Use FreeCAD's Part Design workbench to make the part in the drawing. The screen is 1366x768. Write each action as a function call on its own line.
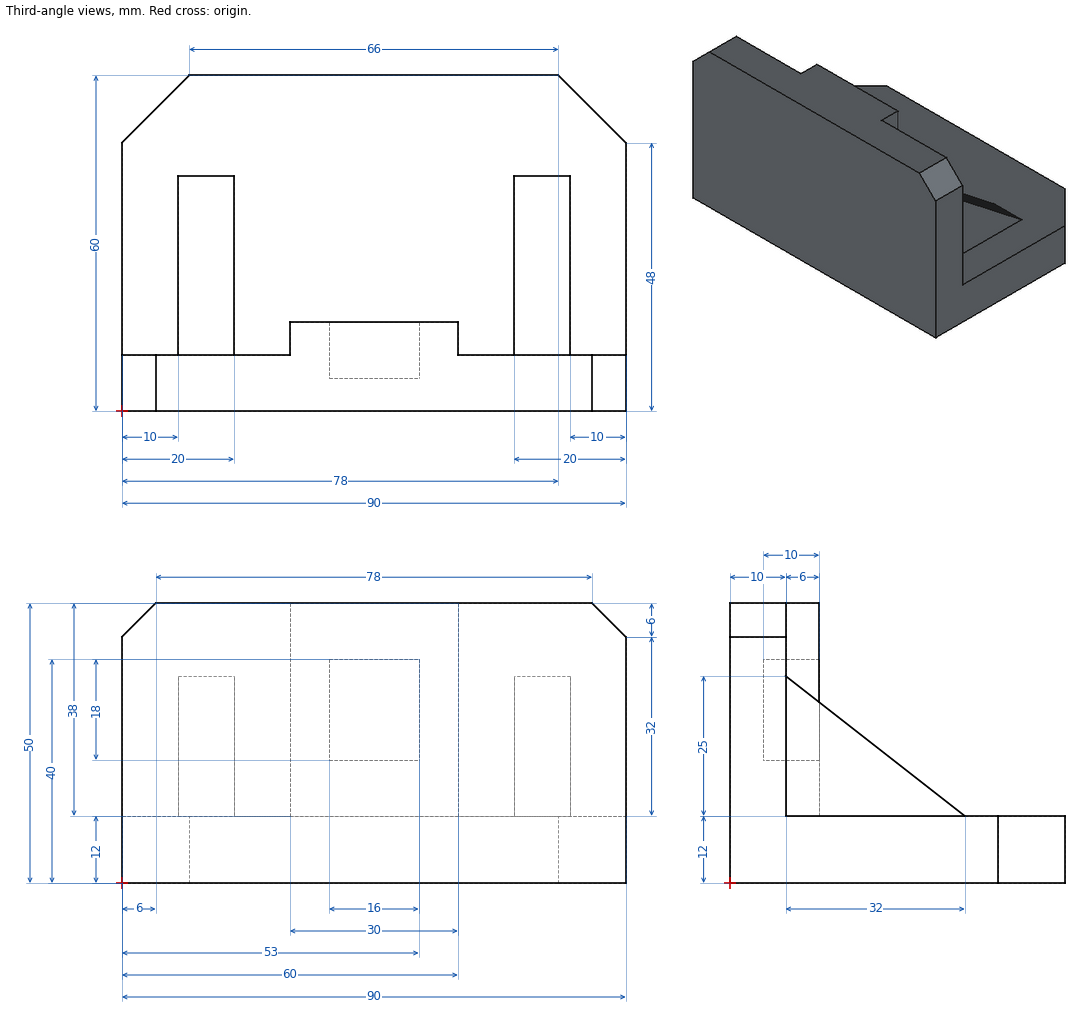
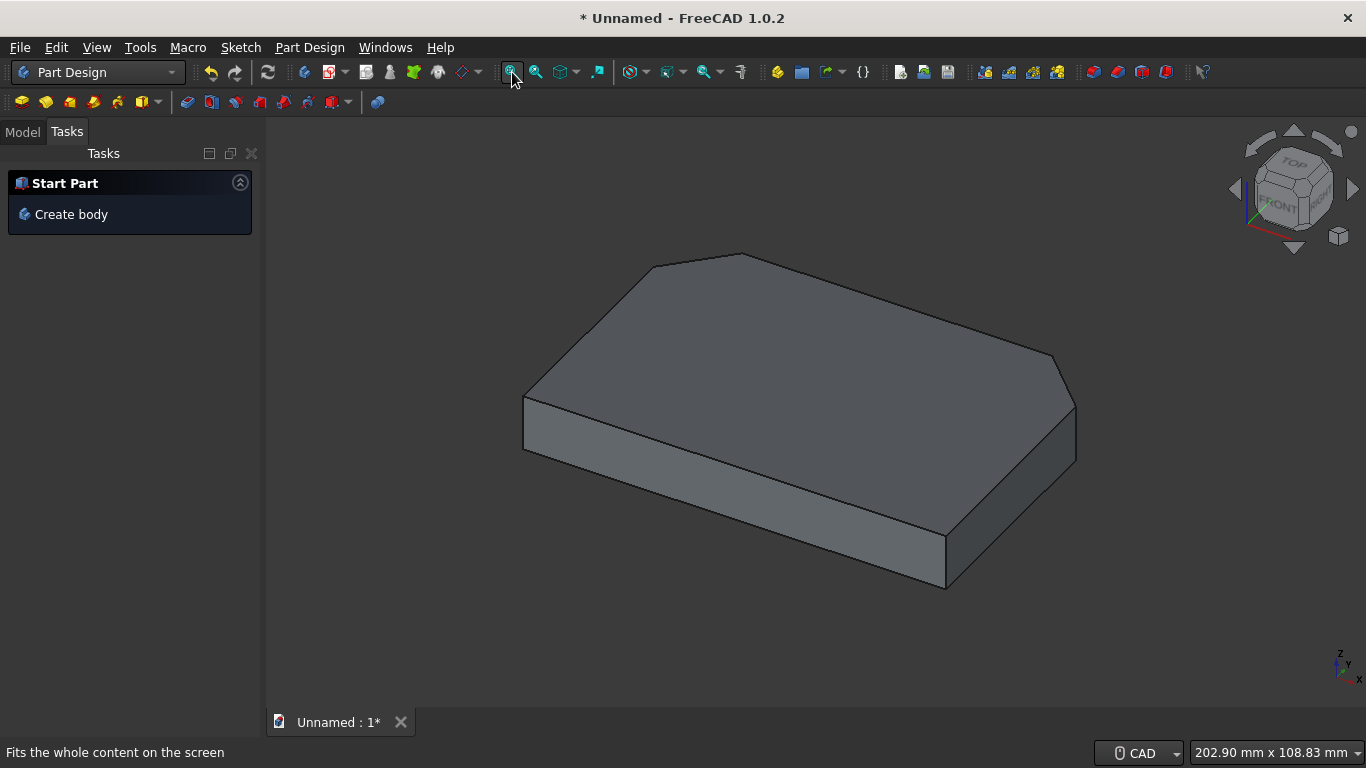
click(330, 72)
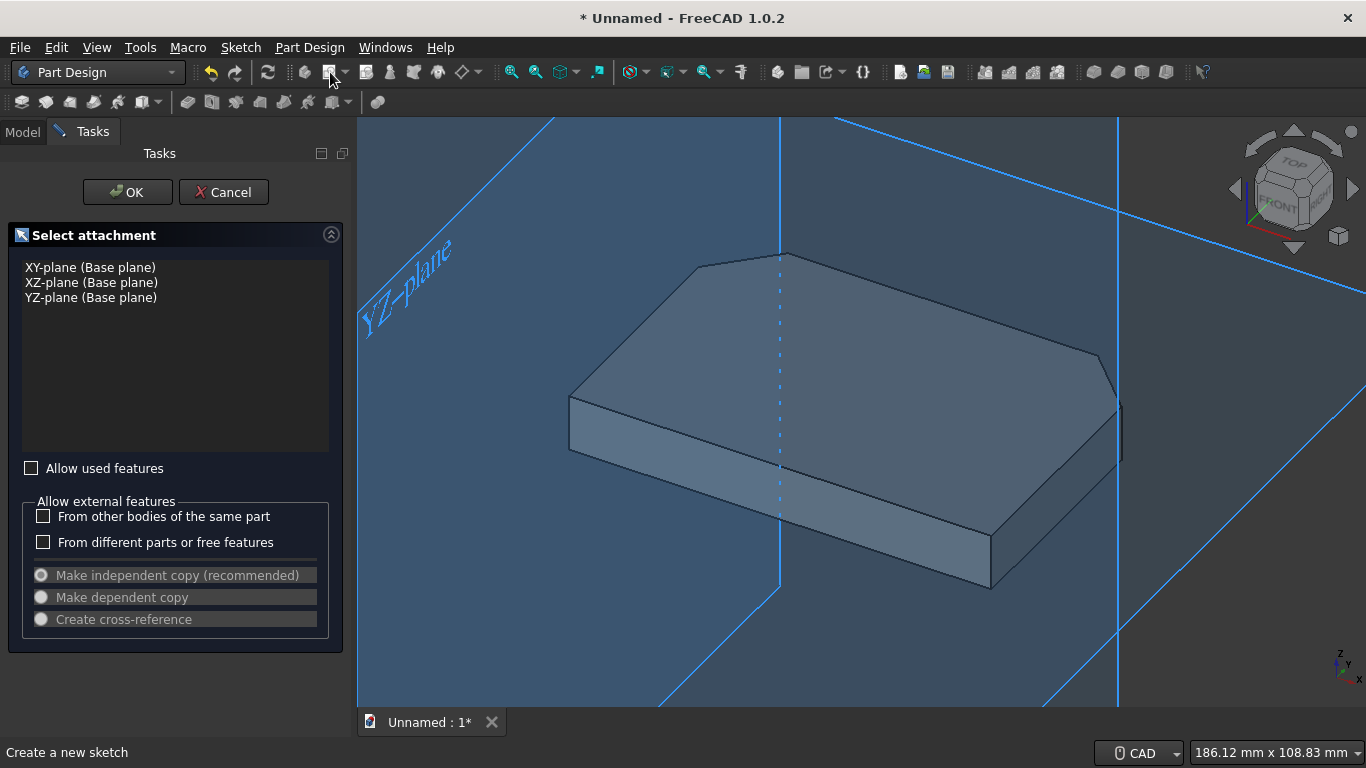
click(82, 282)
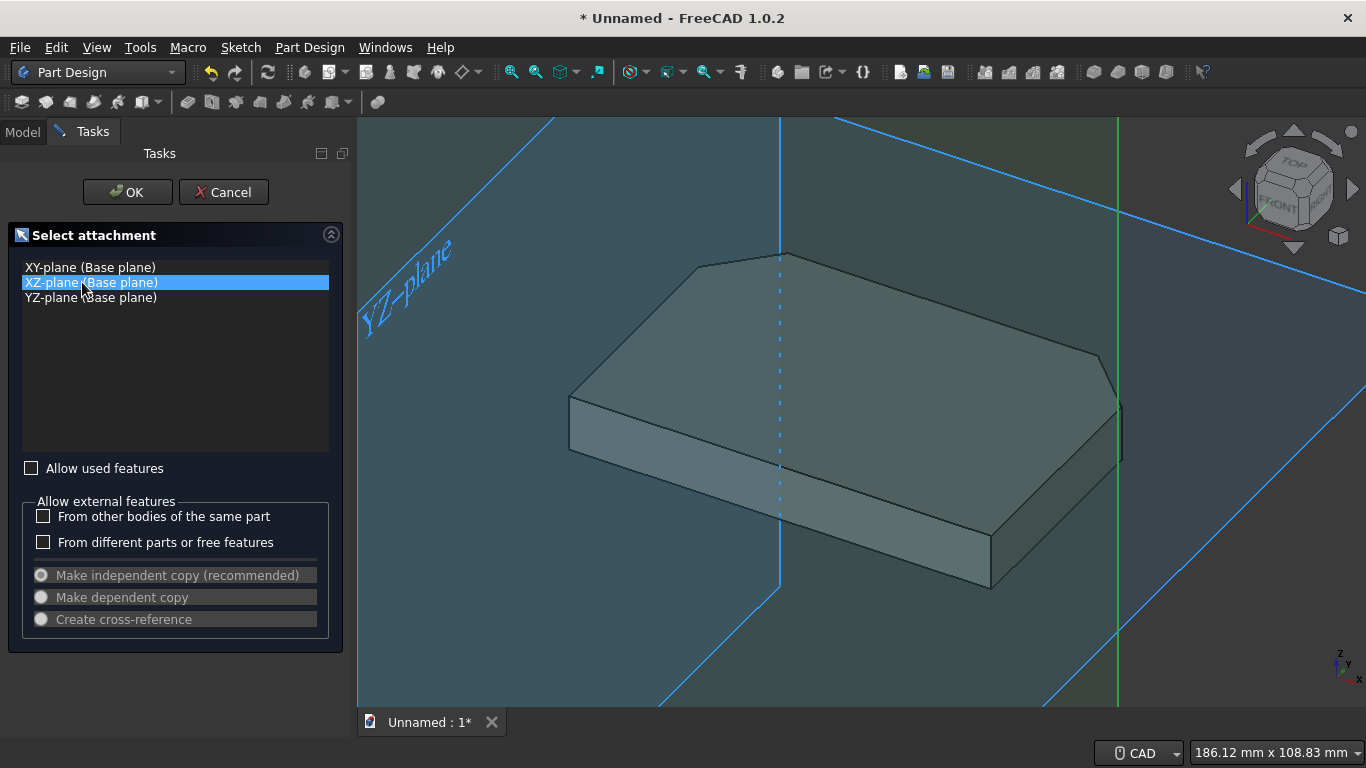
click(128, 192)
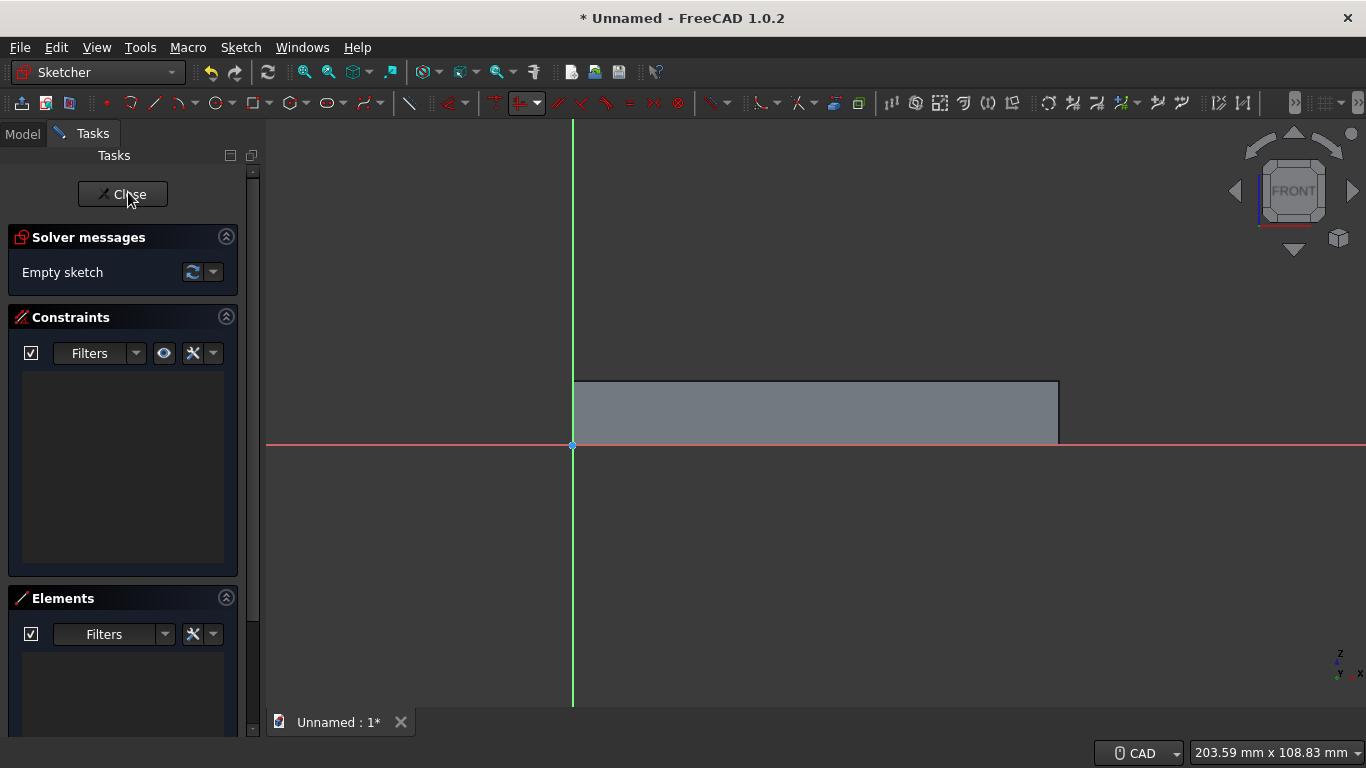
click(132, 104)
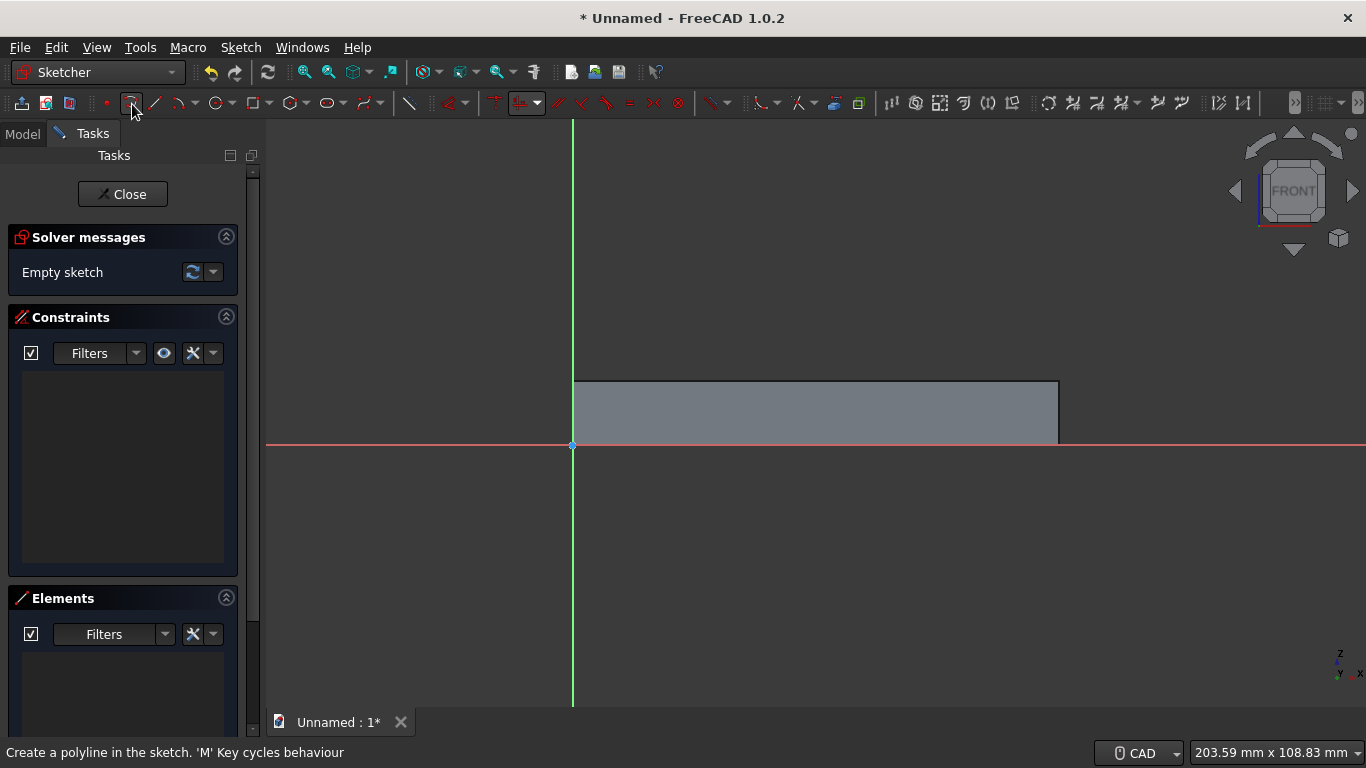
click(573, 381)
click(1059, 381)
click(1059, 208)
click(1027, 175)
click(605, 175)
click(582, 208)
click(573, 382)
key(Escape)
key(Escape)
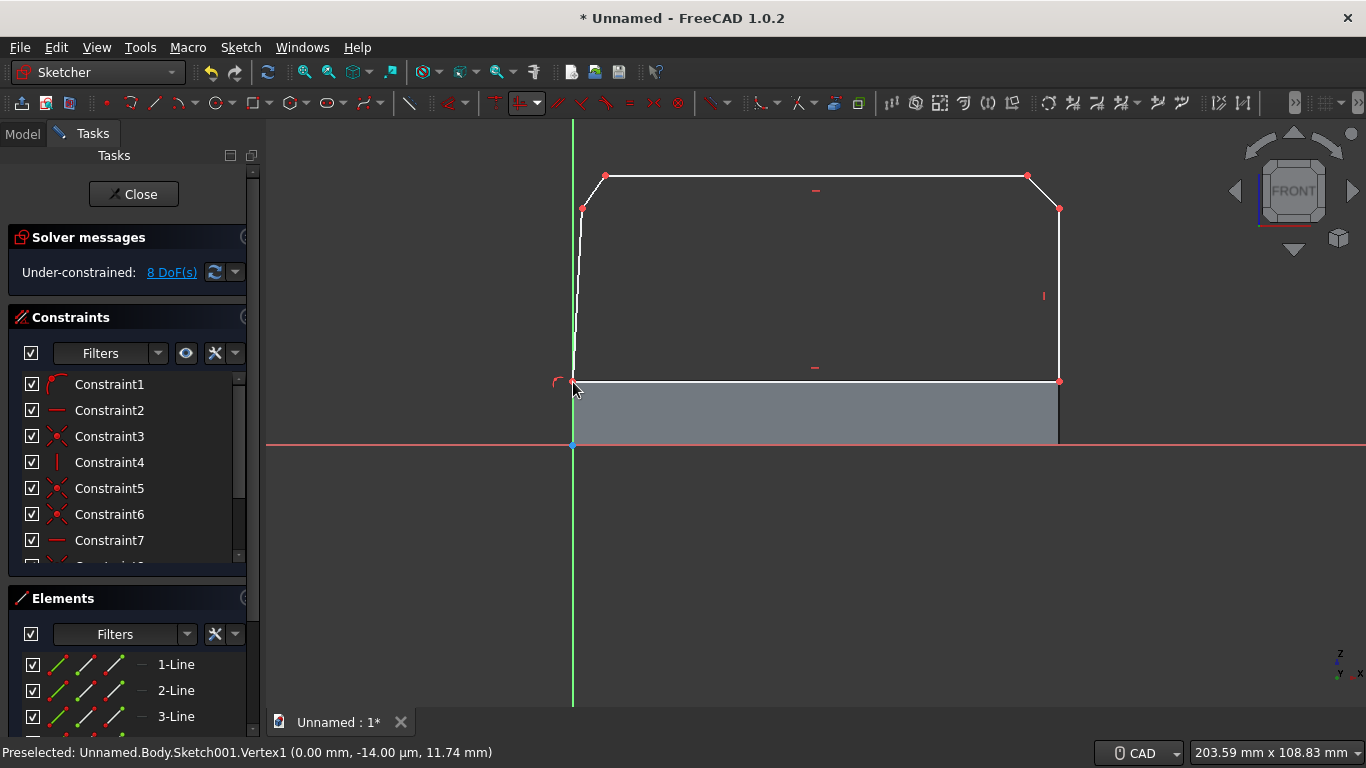
click(576, 330)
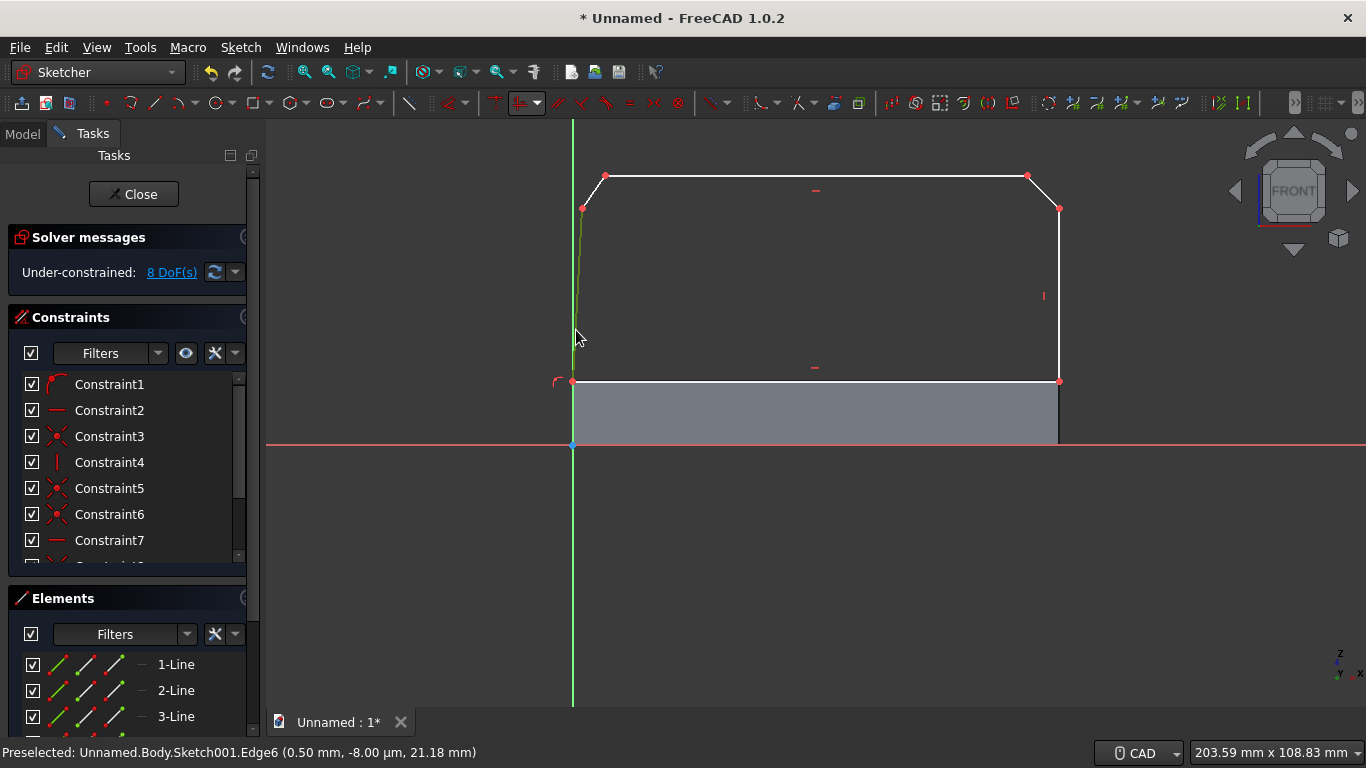
key(v)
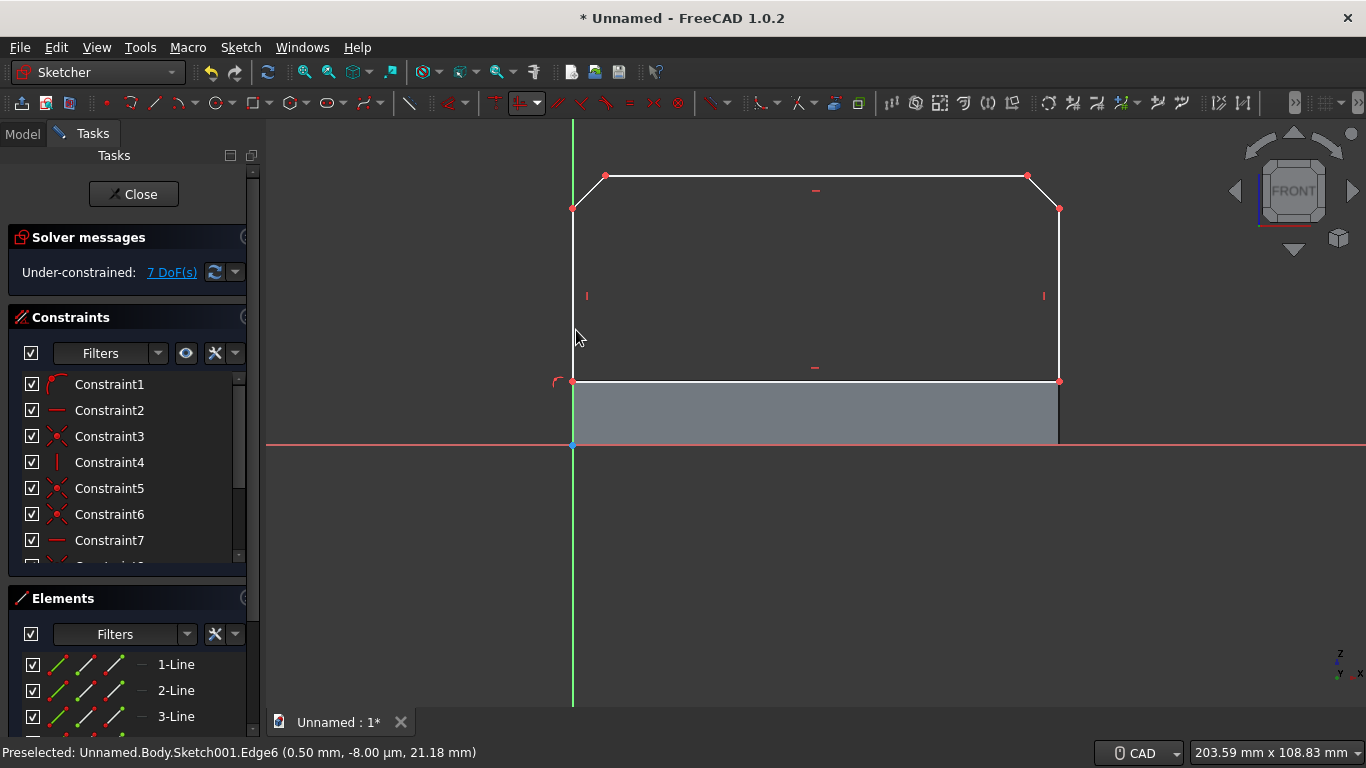
click(448, 104)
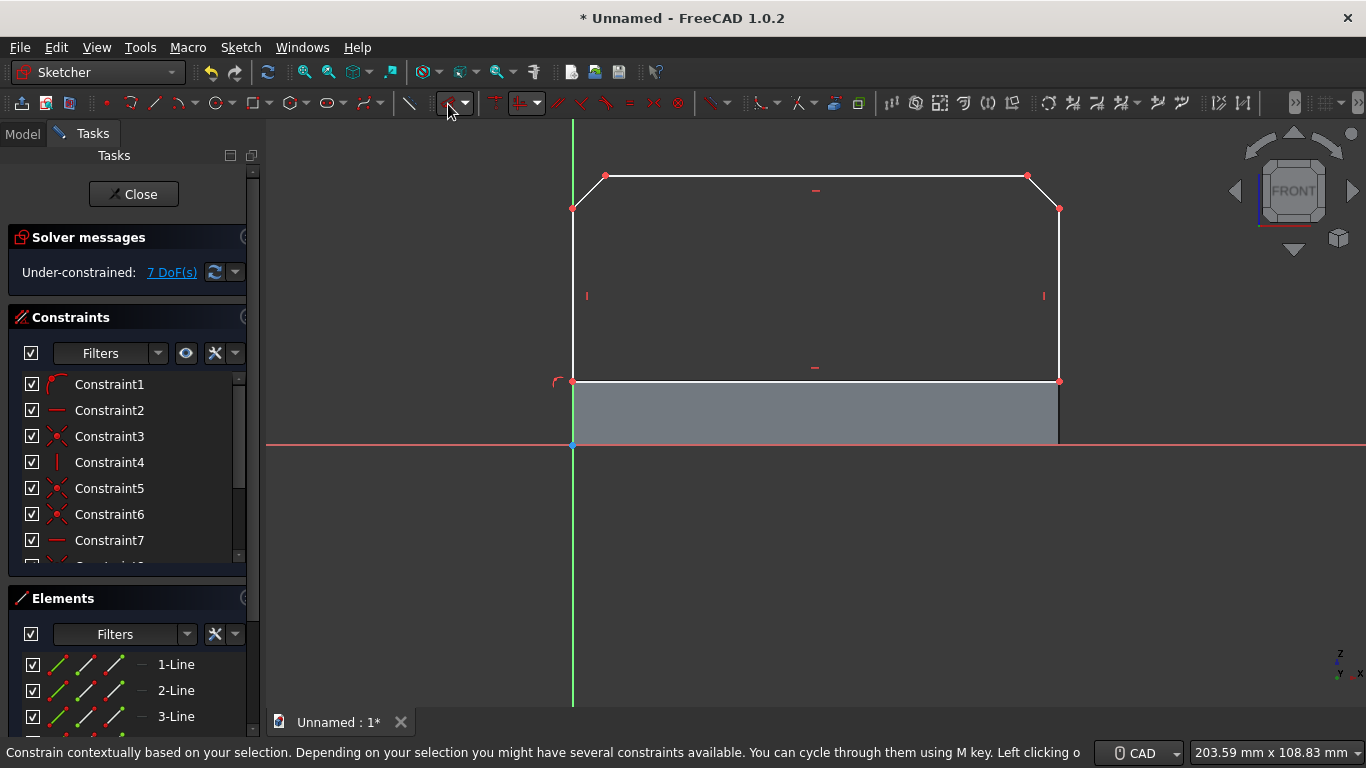
click(719, 382)
click(816, 416)